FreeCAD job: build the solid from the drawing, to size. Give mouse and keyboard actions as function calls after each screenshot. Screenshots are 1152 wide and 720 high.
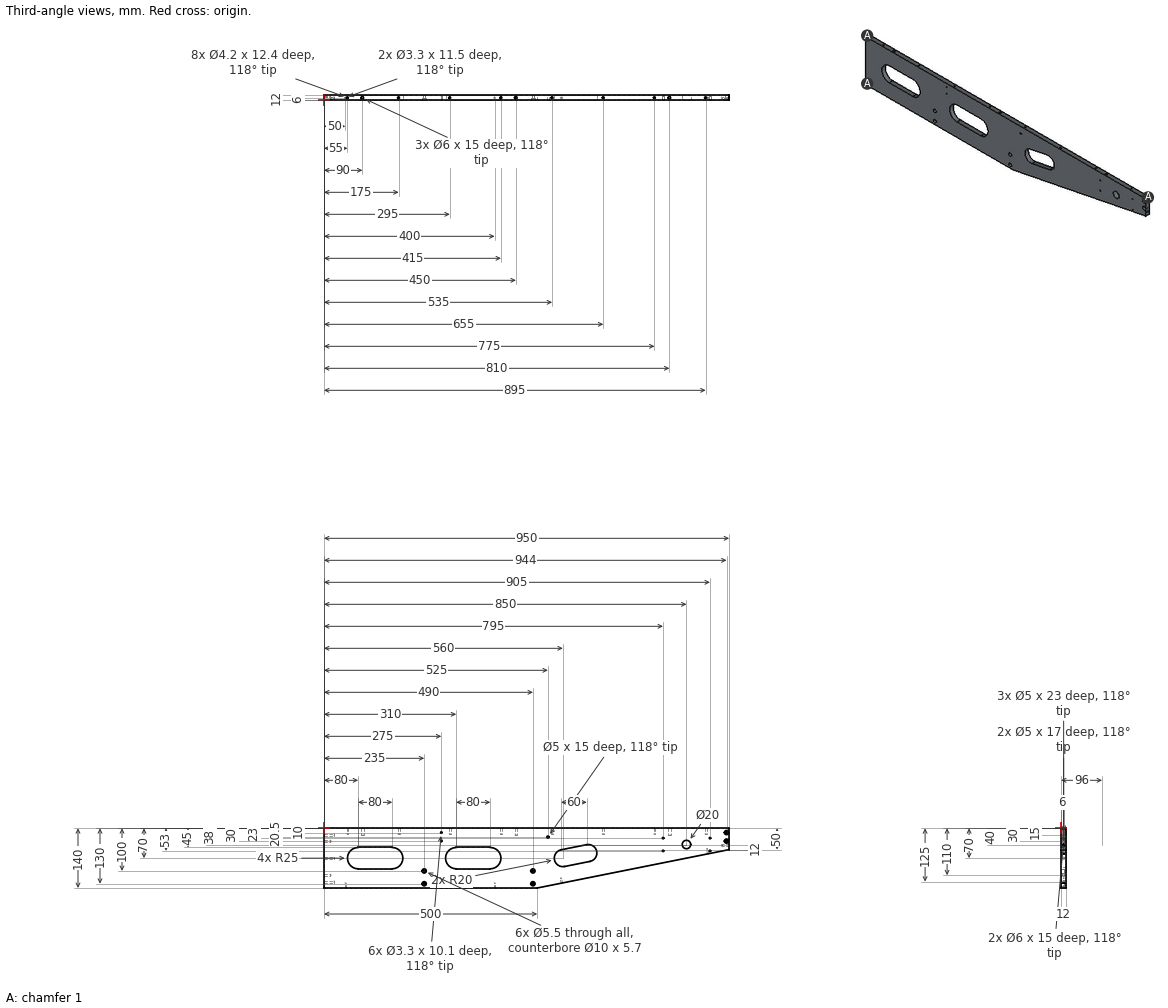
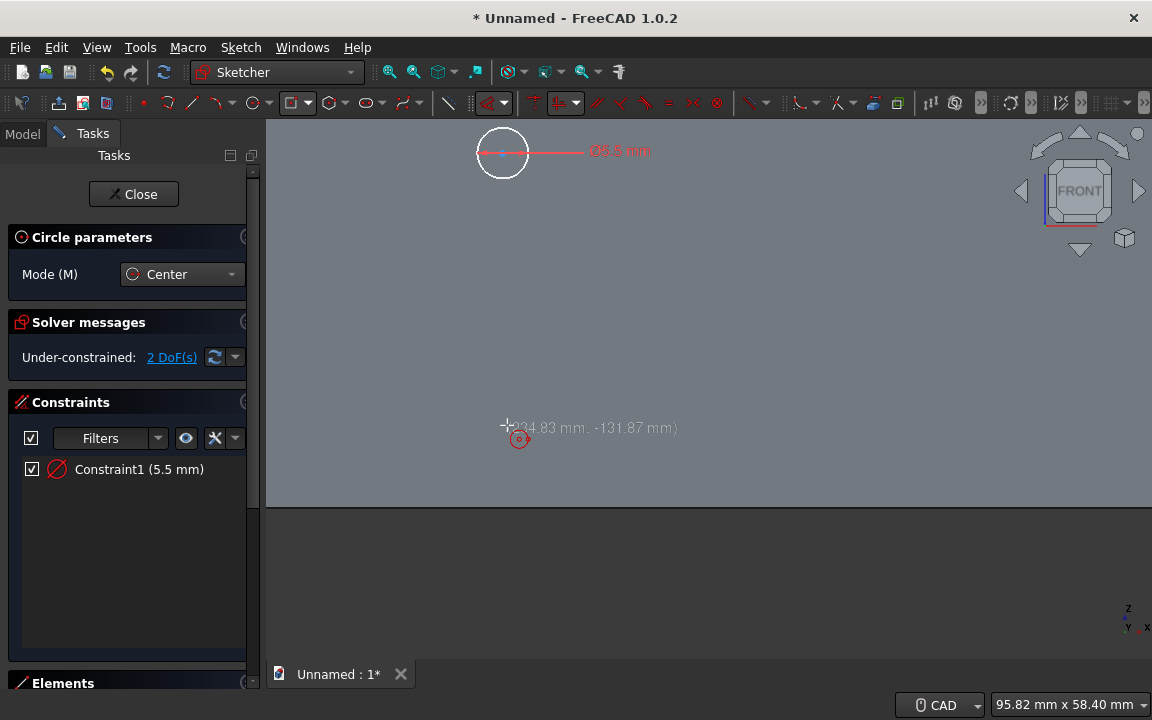
scroll(507, 425, down, 14)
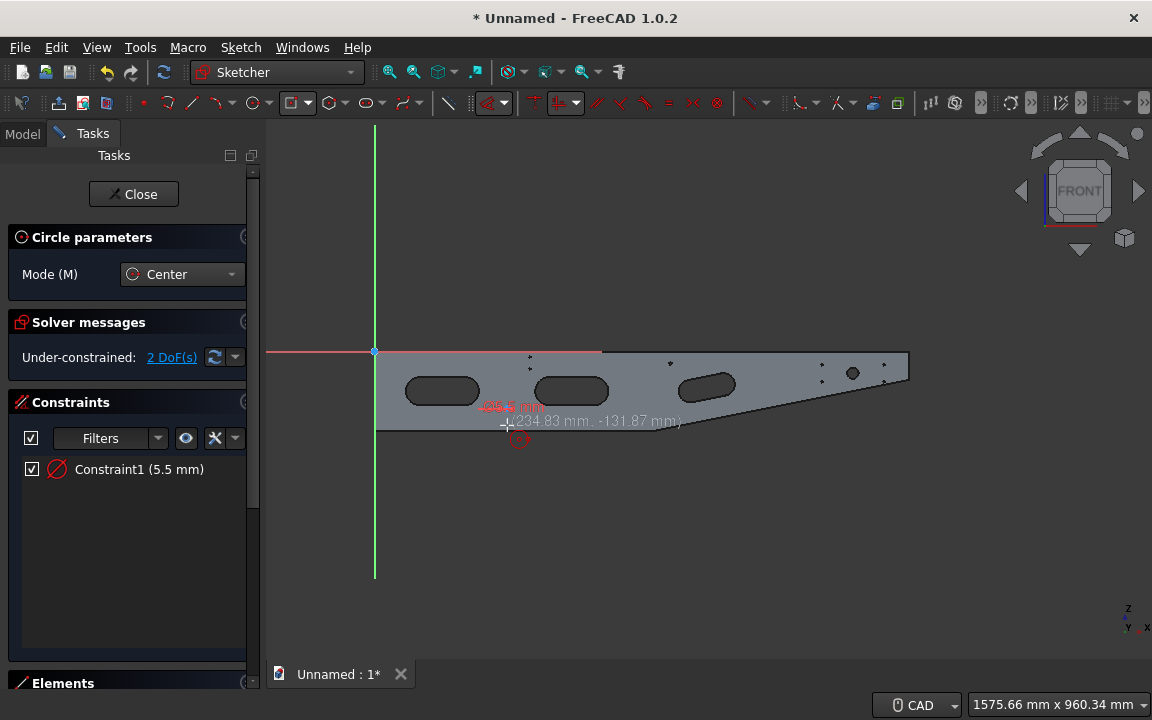
click(507, 425)
move(508, 424)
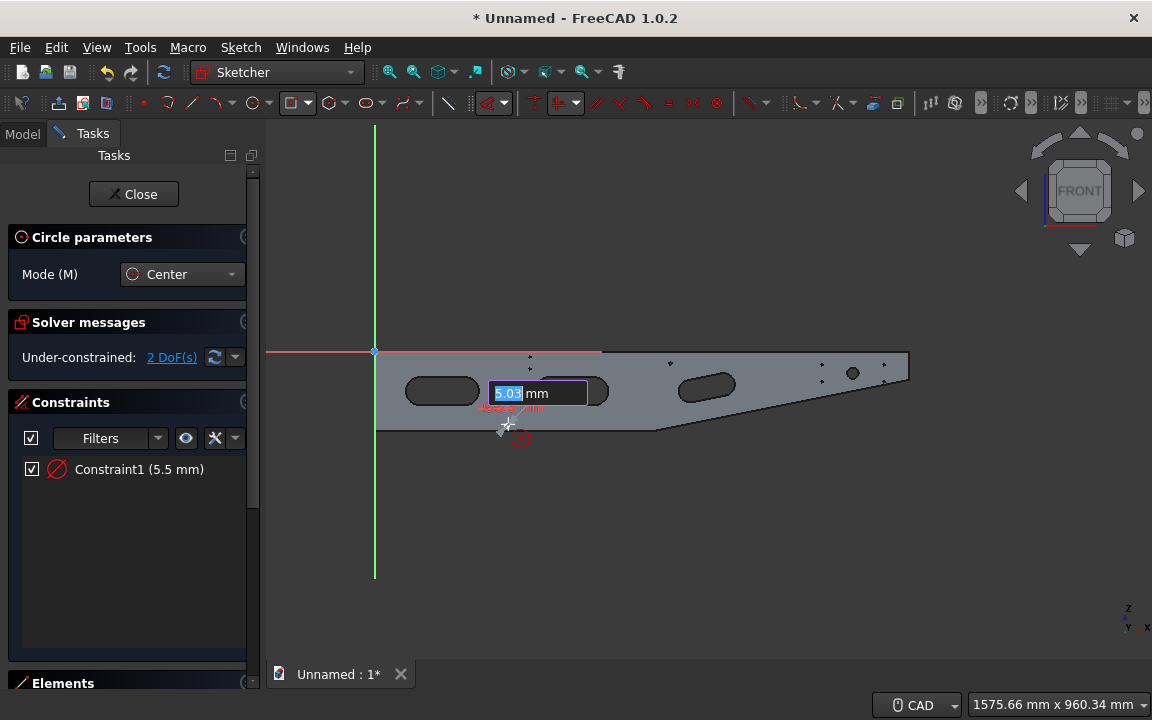
text(5.5)
key(Return)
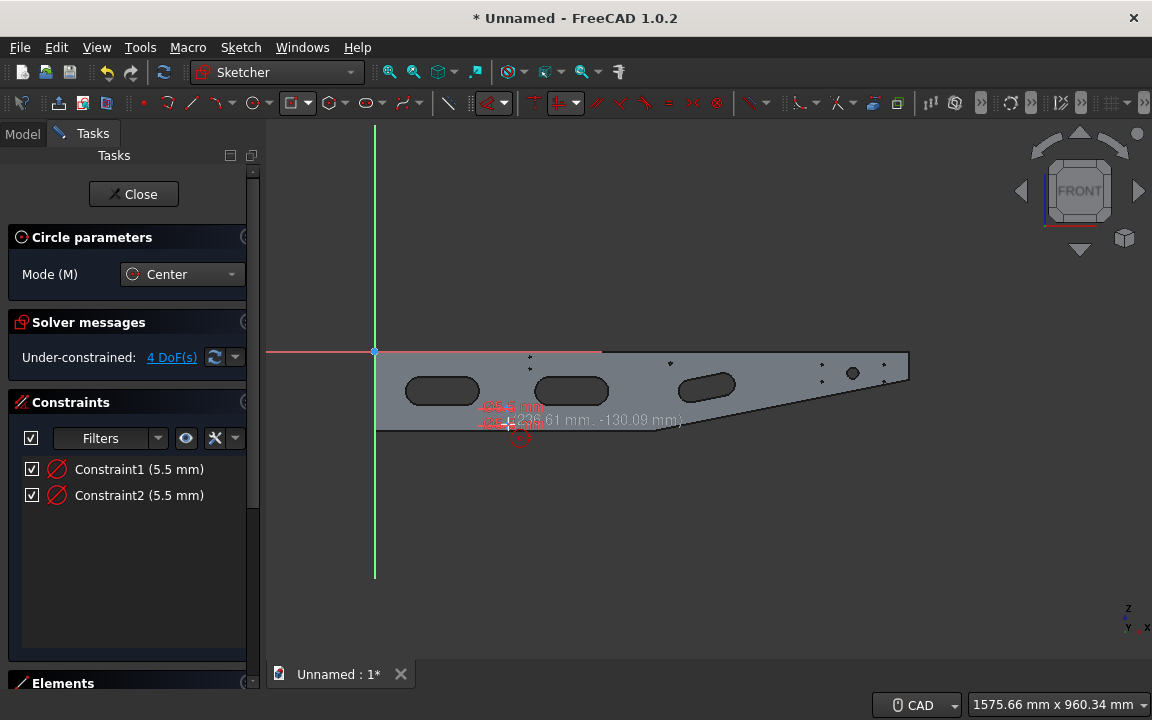
scroll(650, 408, up, 14)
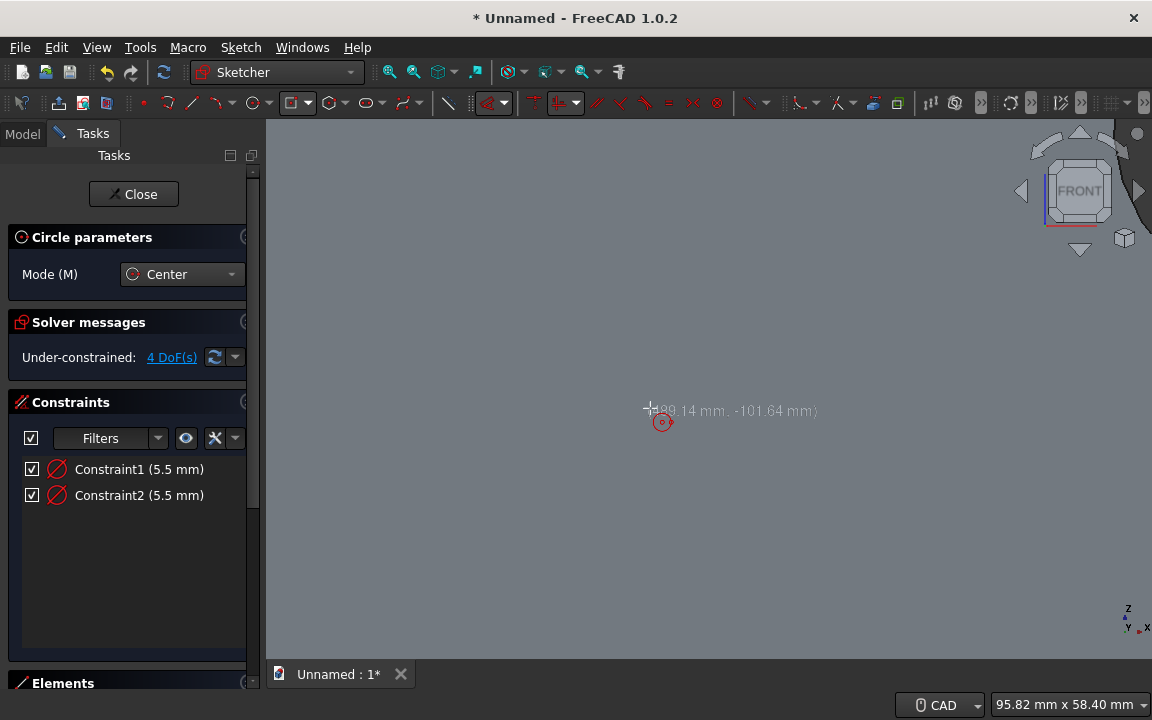
scroll(650, 408, down, 14)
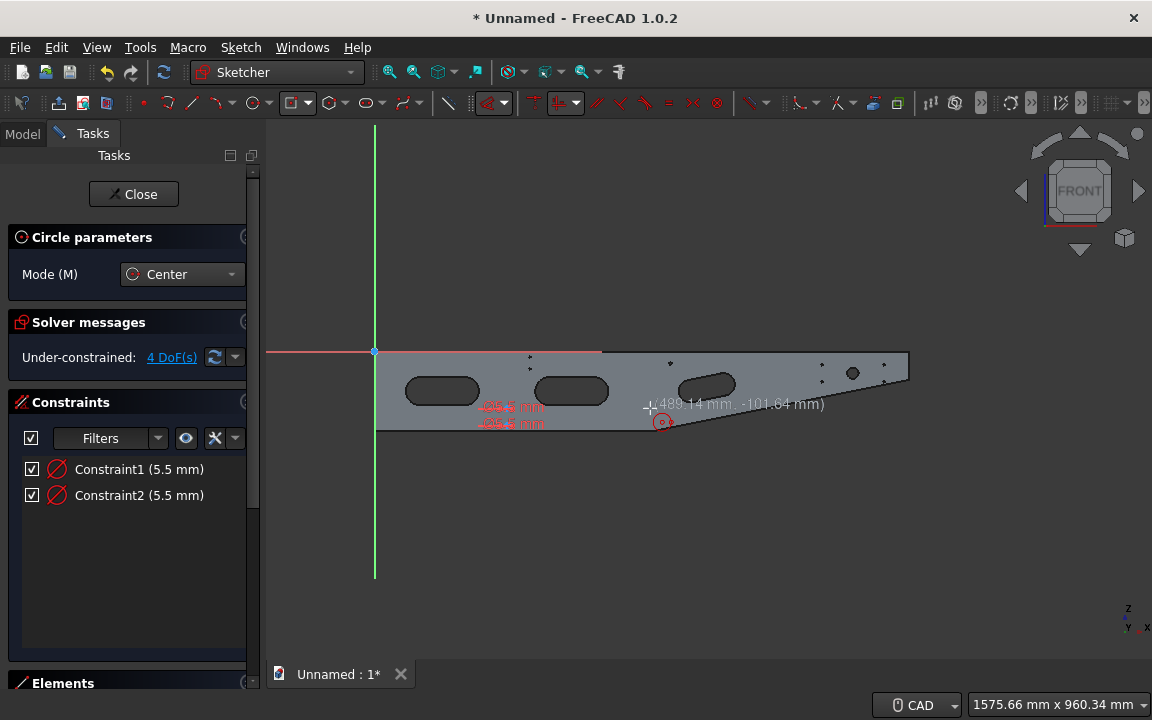
click(650, 408)
move(652, 407)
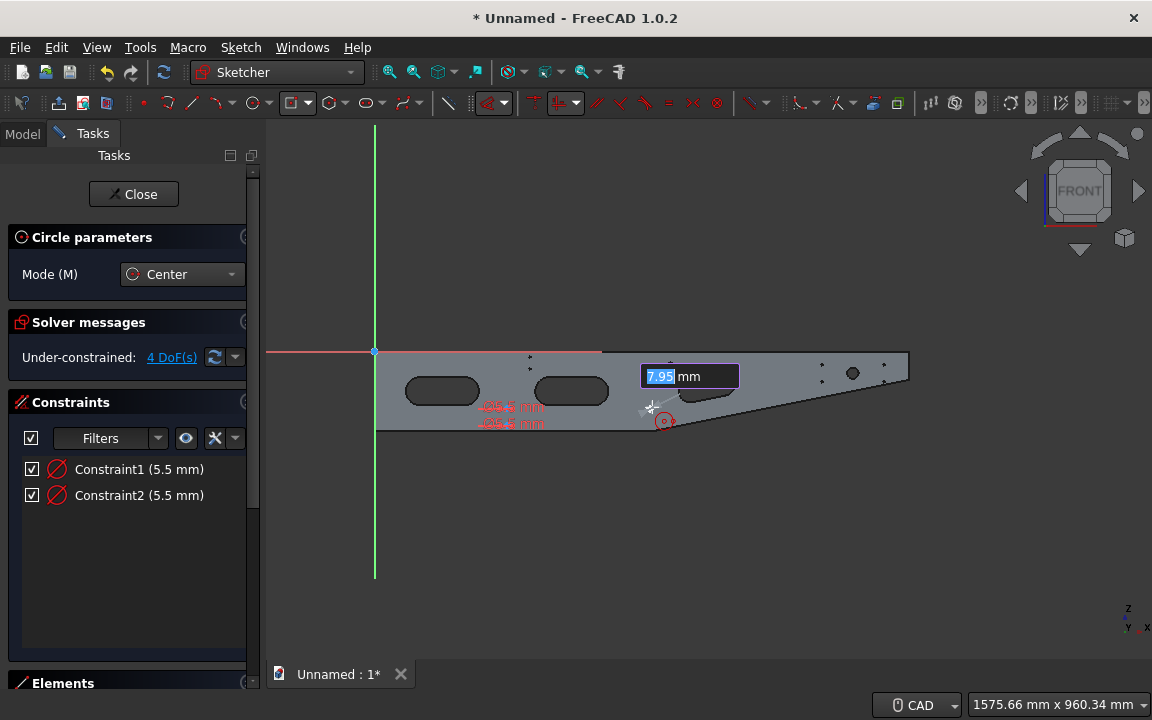
text(5.5)
key(Return)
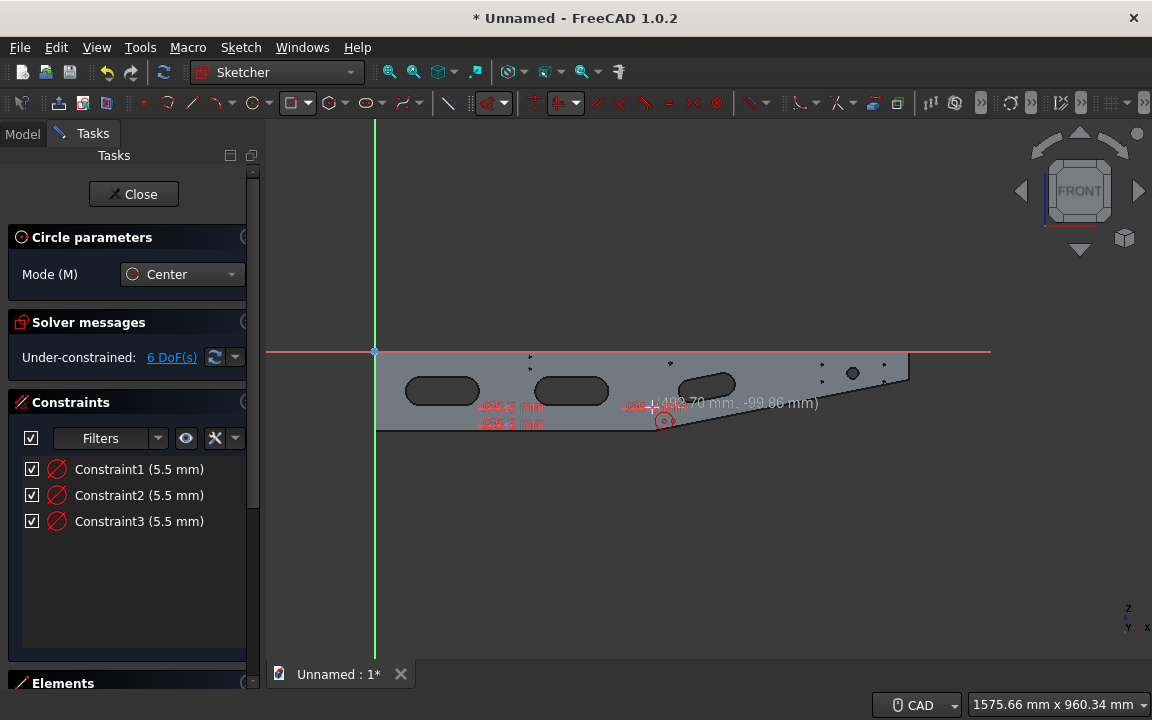
scroll(650, 425, up, 14)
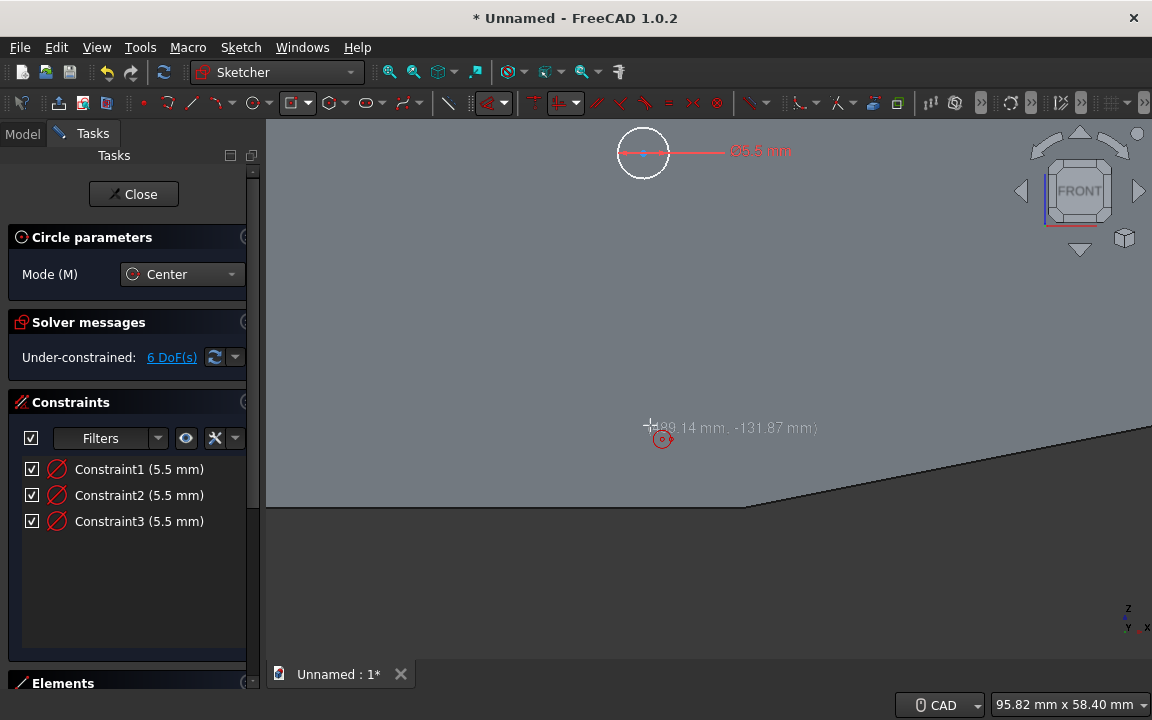
scroll(650, 425, down, 14)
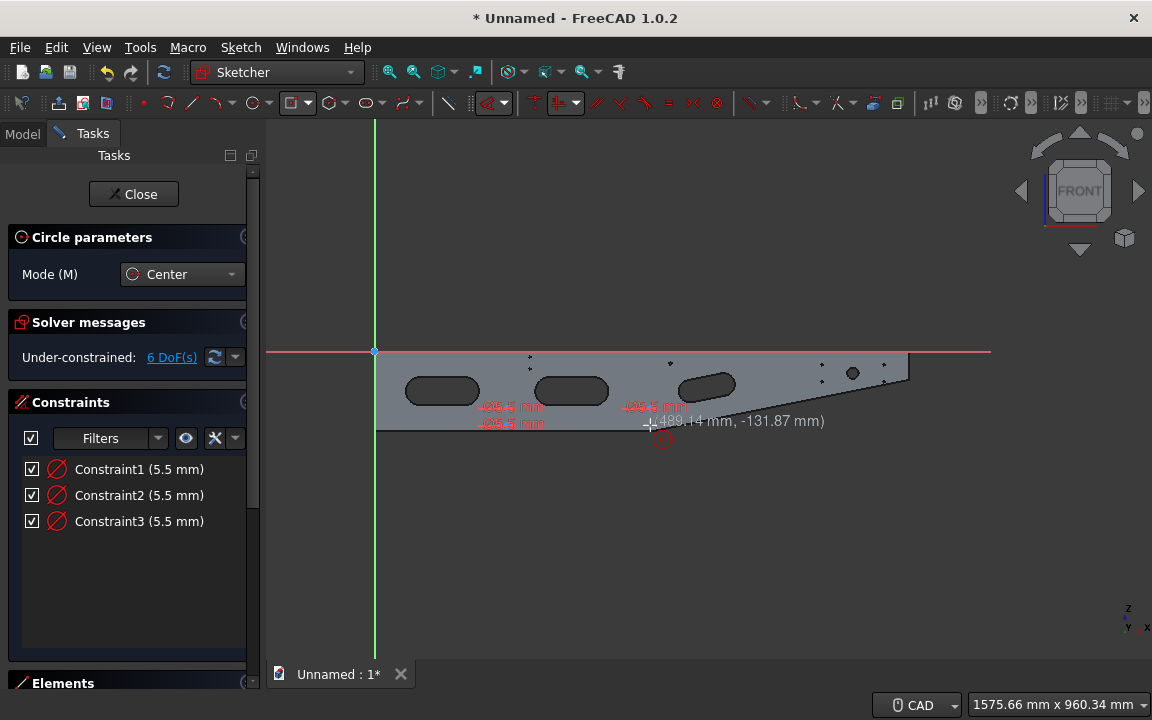
click(650, 425)
move(652, 424)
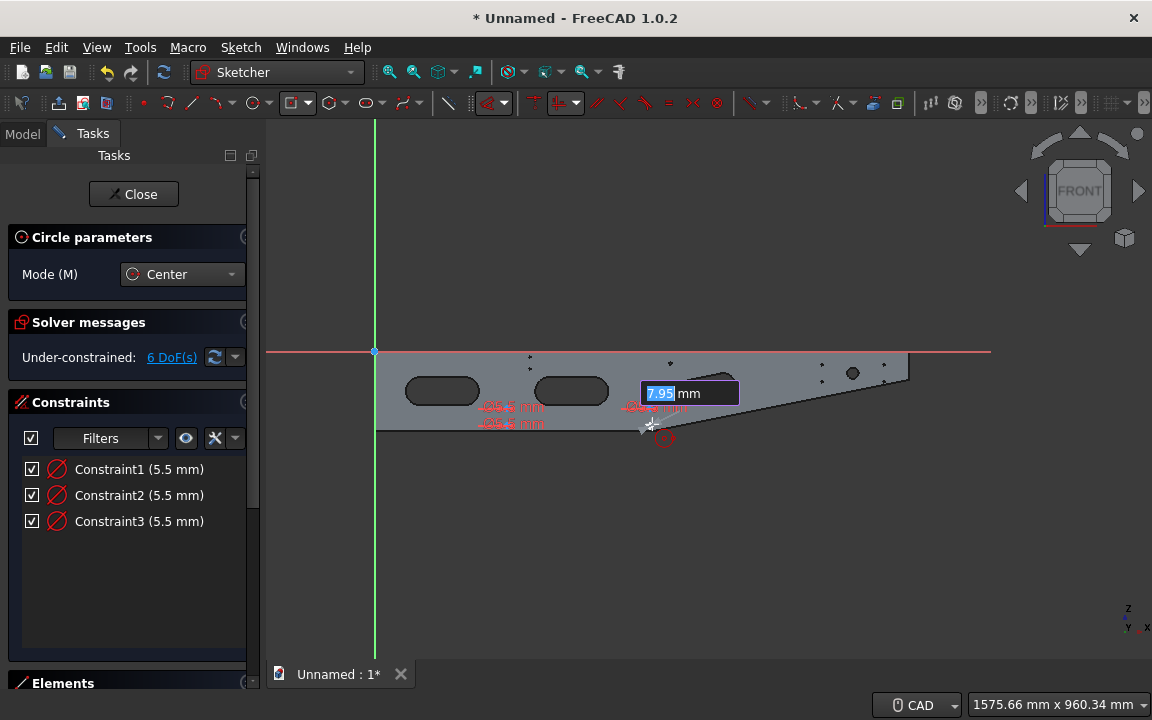
text(5.5)
key(Return)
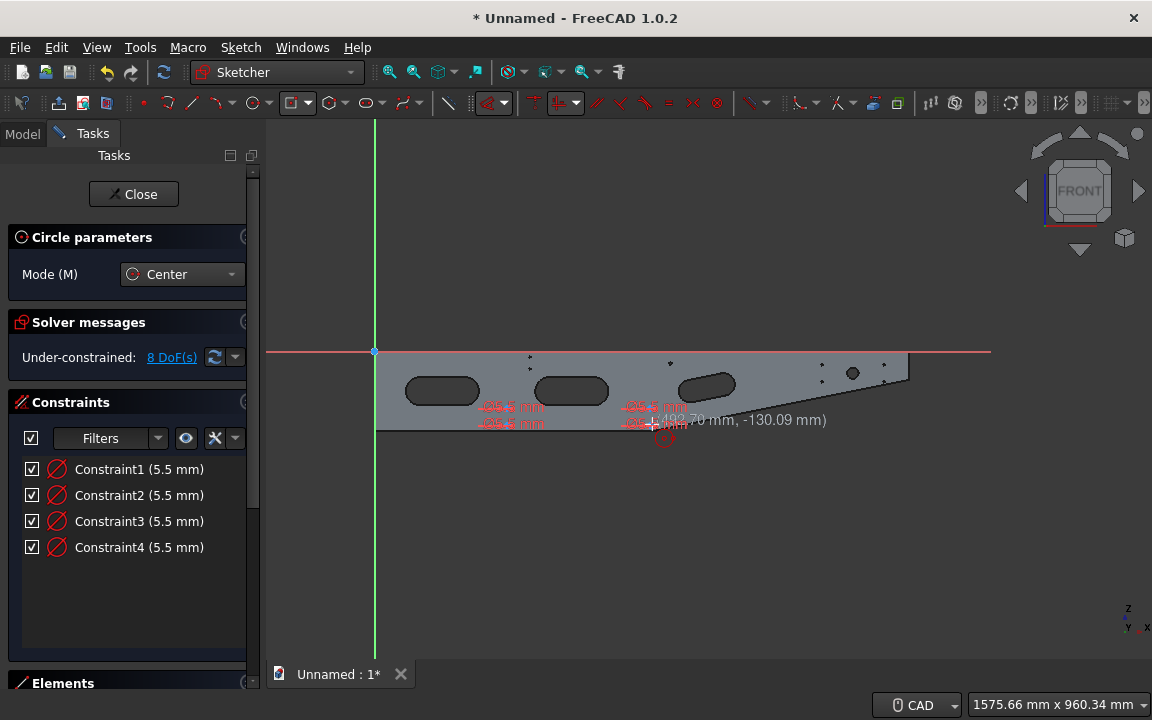
scroll(906, 357, up, 14)